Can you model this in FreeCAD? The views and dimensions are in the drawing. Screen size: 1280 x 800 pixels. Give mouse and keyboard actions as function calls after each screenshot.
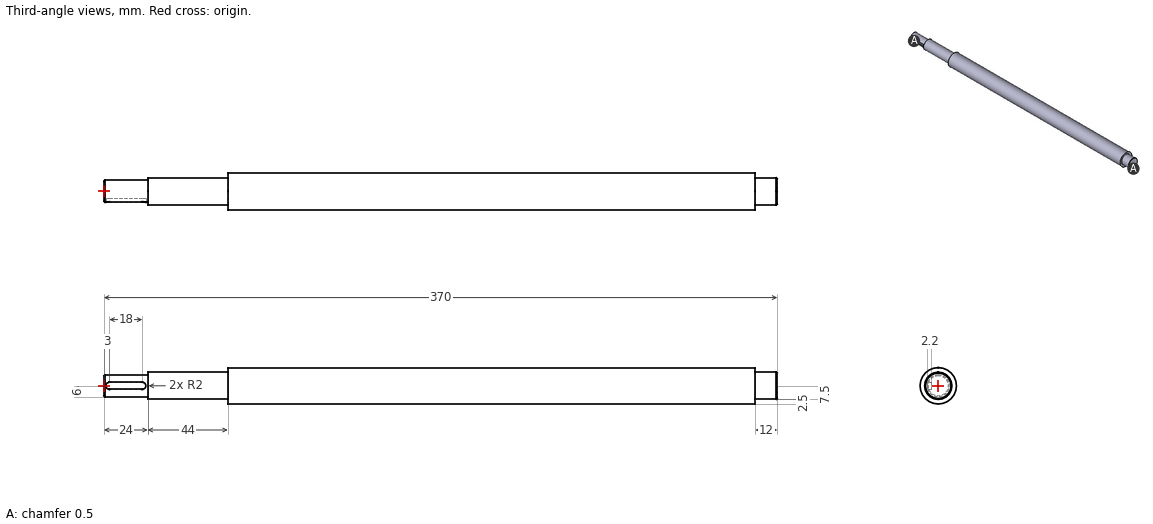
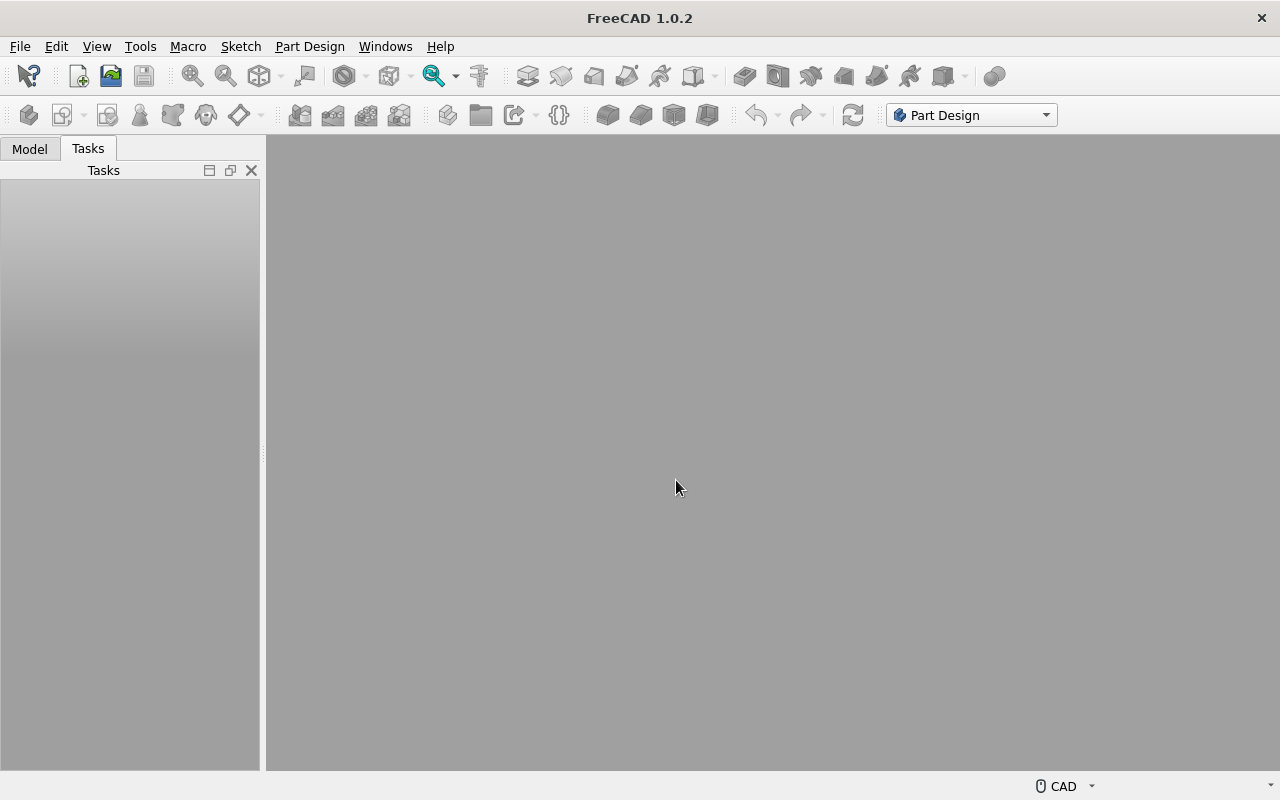
click(78, 76)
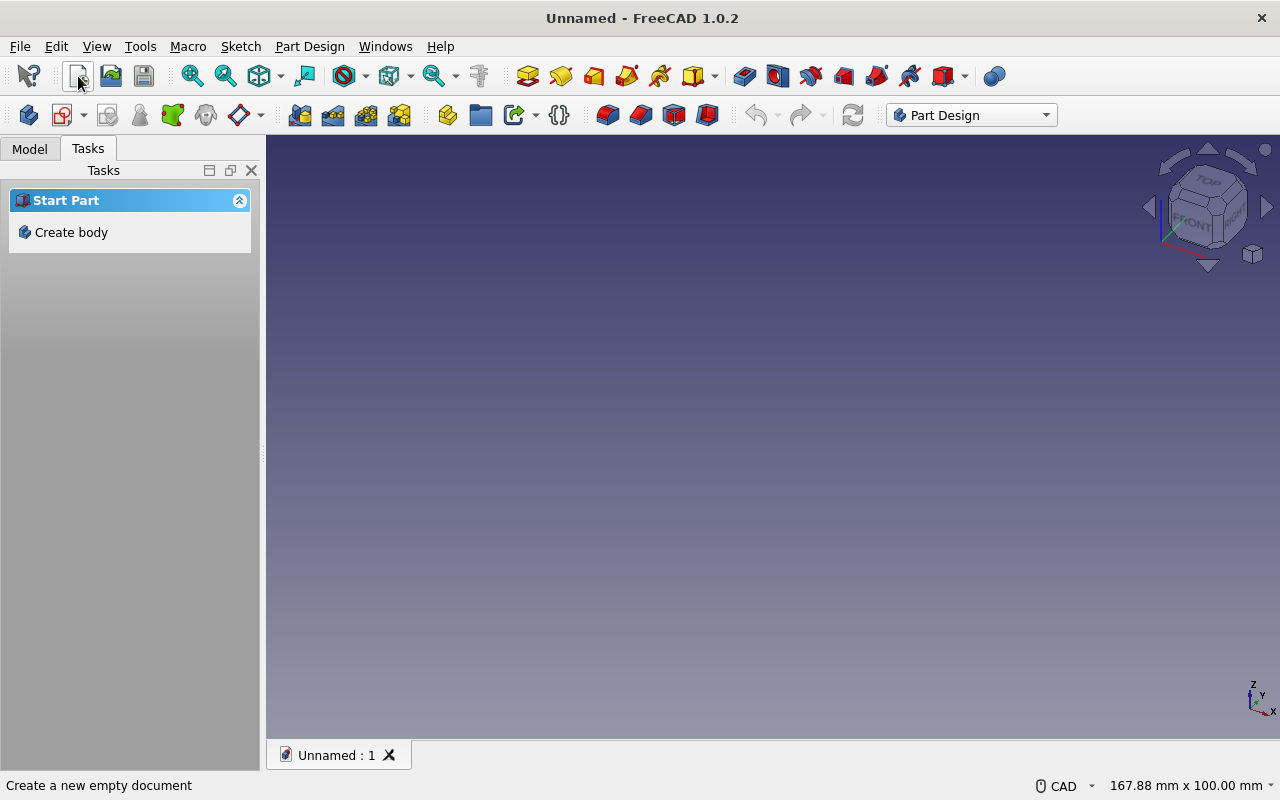
click(62, 116)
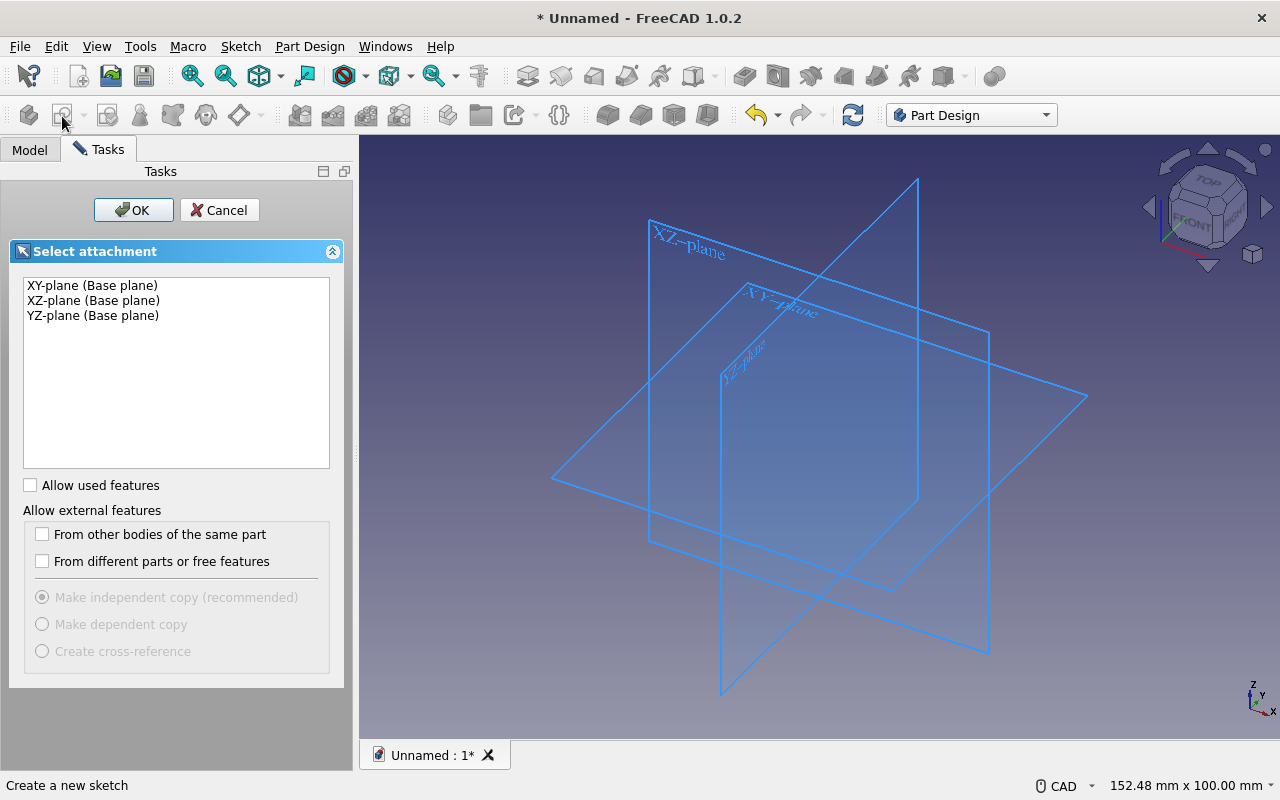
click(84, 300)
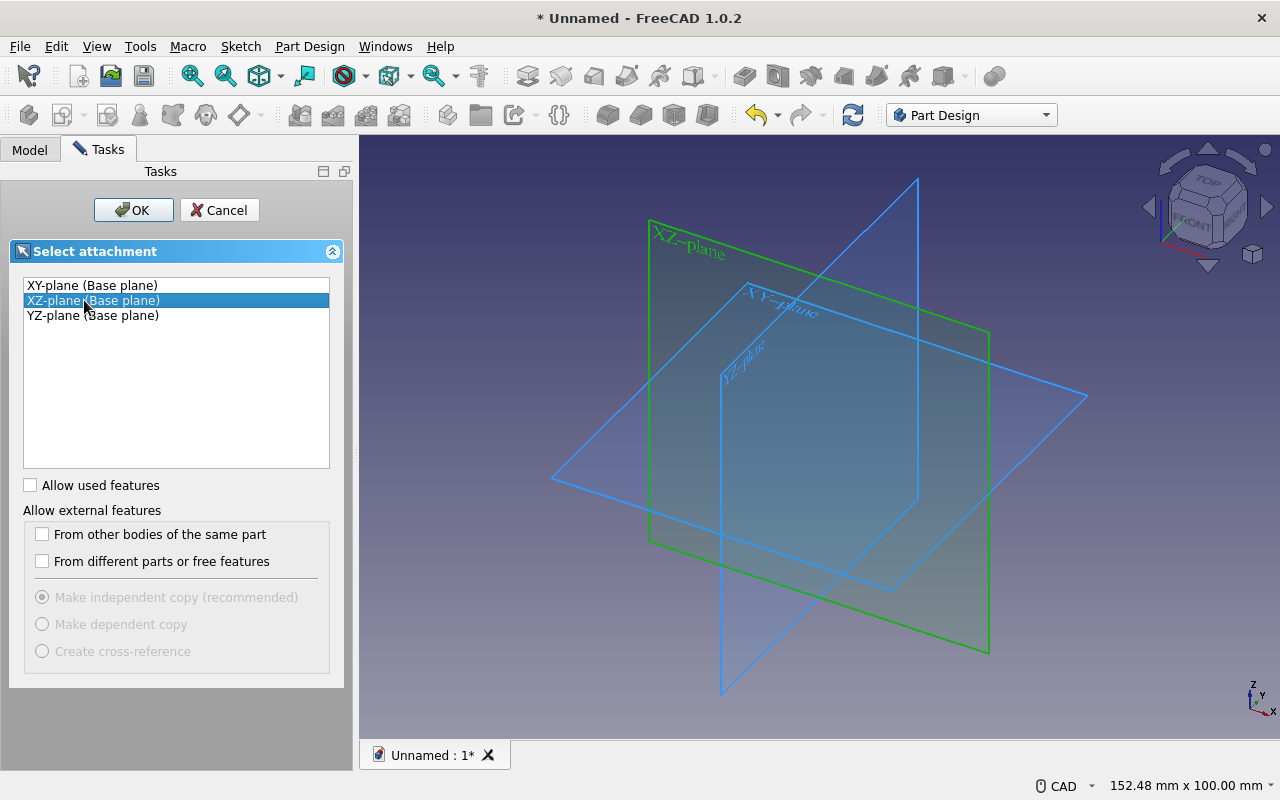
click(134, 210)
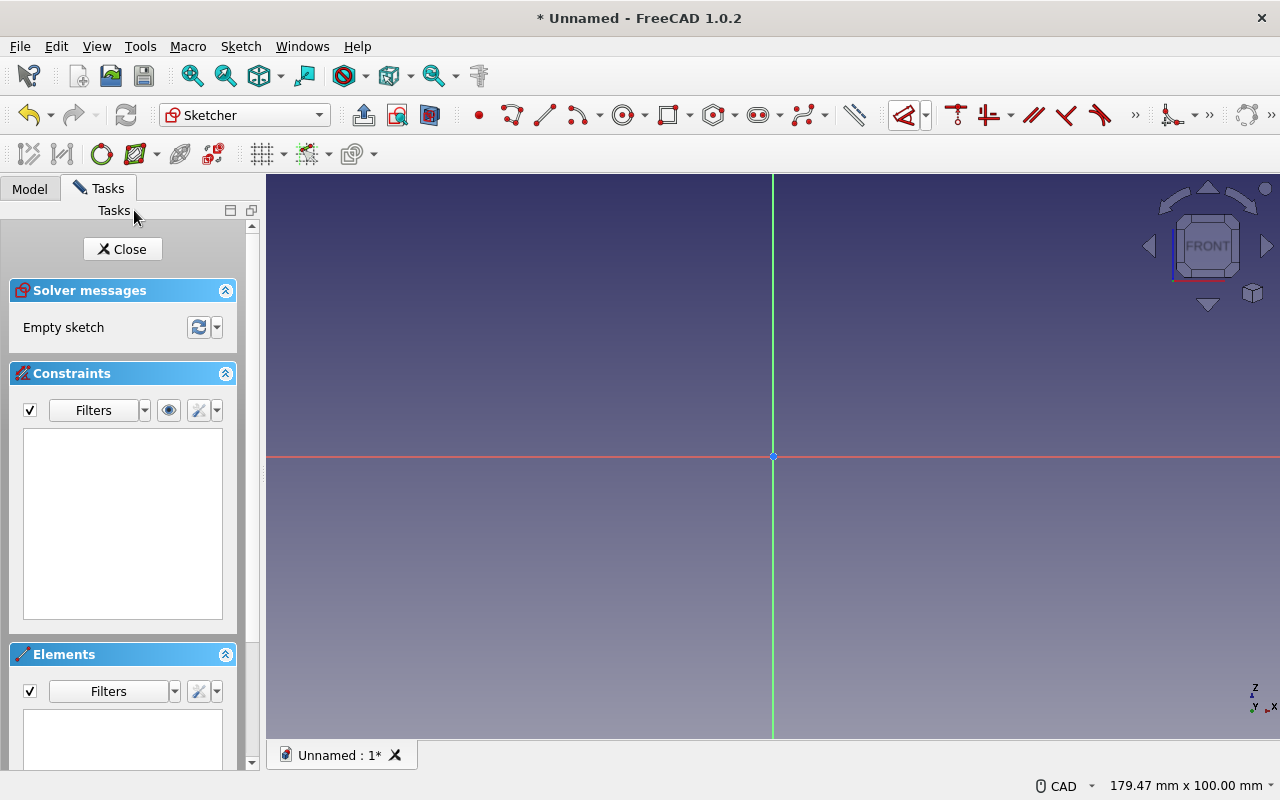
scroll(294, 444, down, 6)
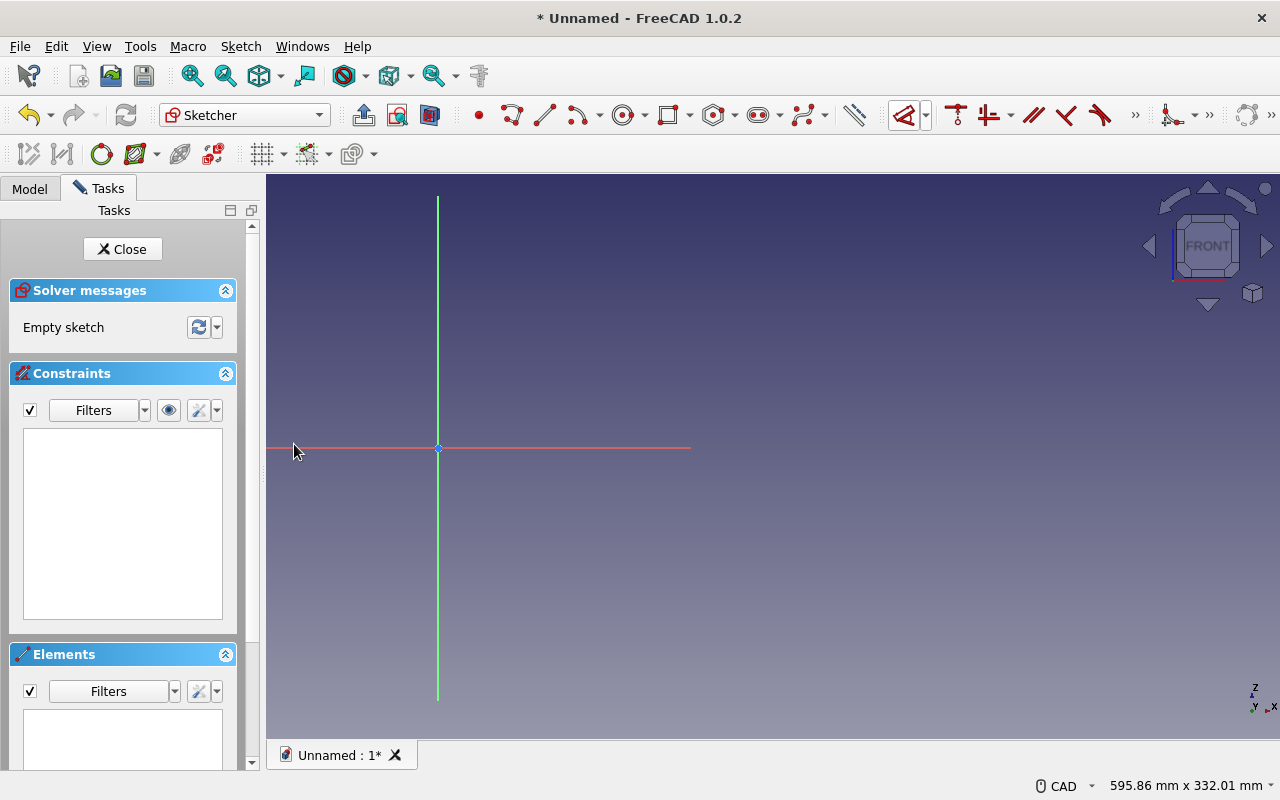
click(512, 116)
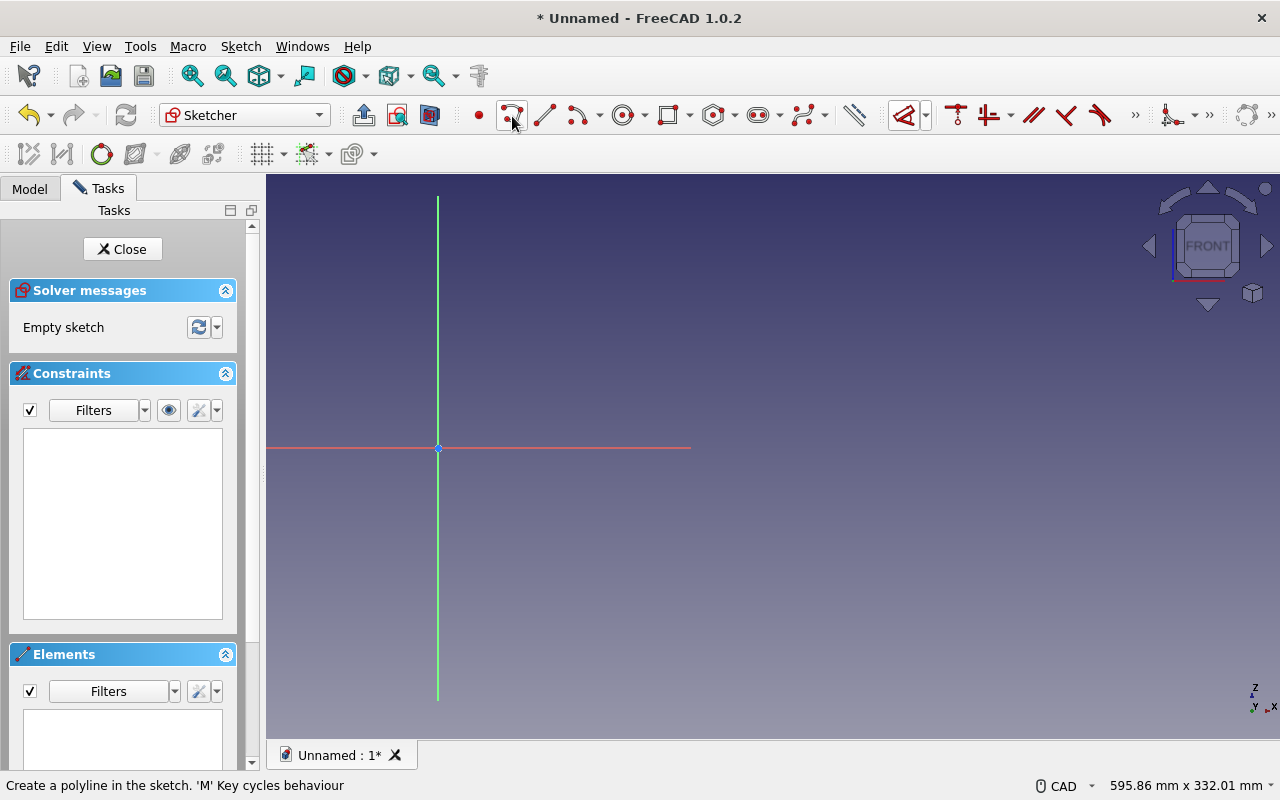
click(438, 448)
click(1068, 457)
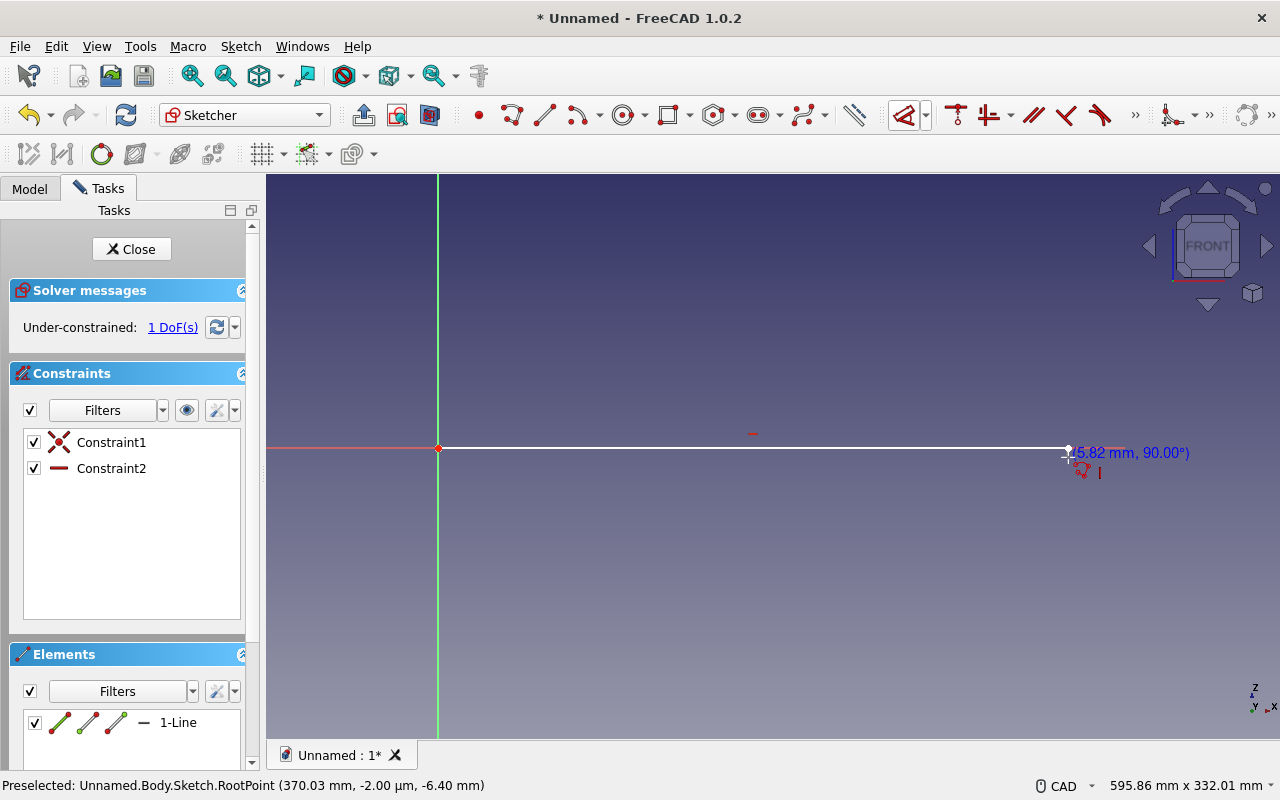
scroll(1068, 461, up, 2)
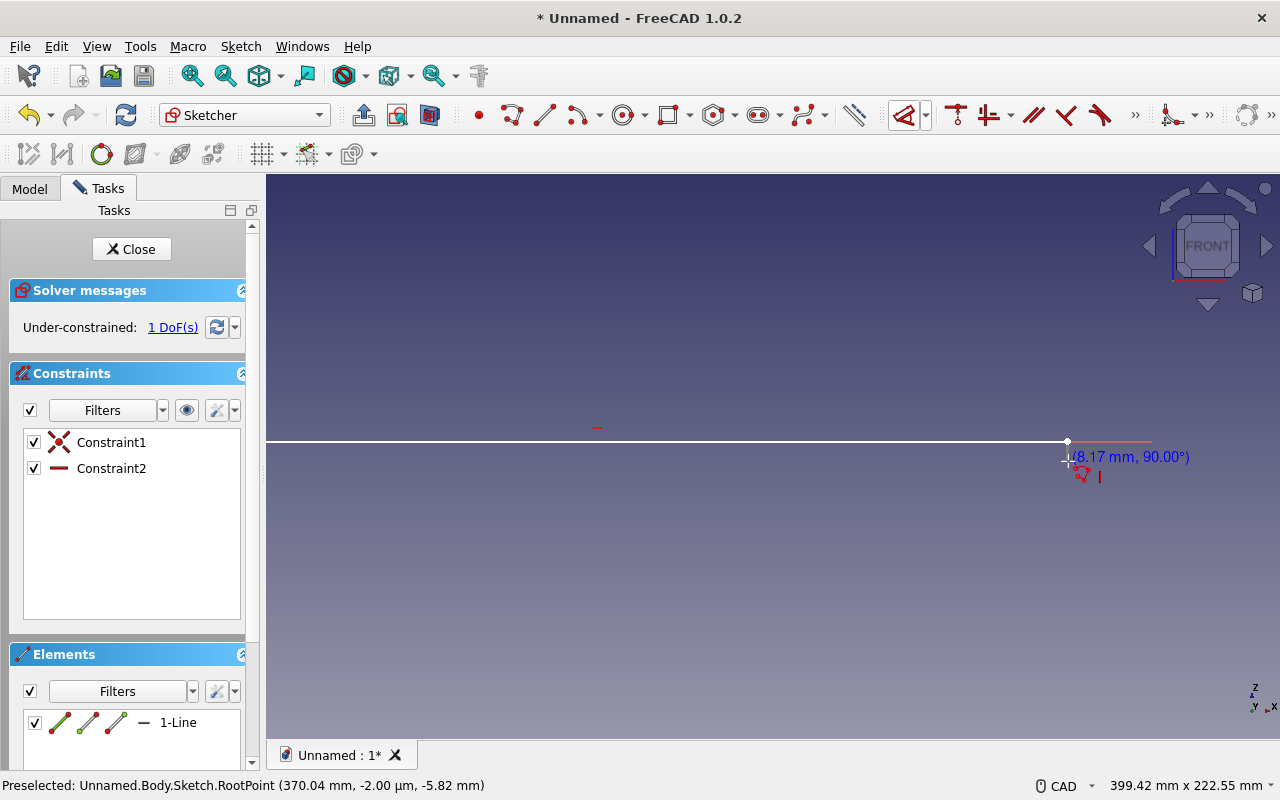
click(1068, 461)
click(1037, 461)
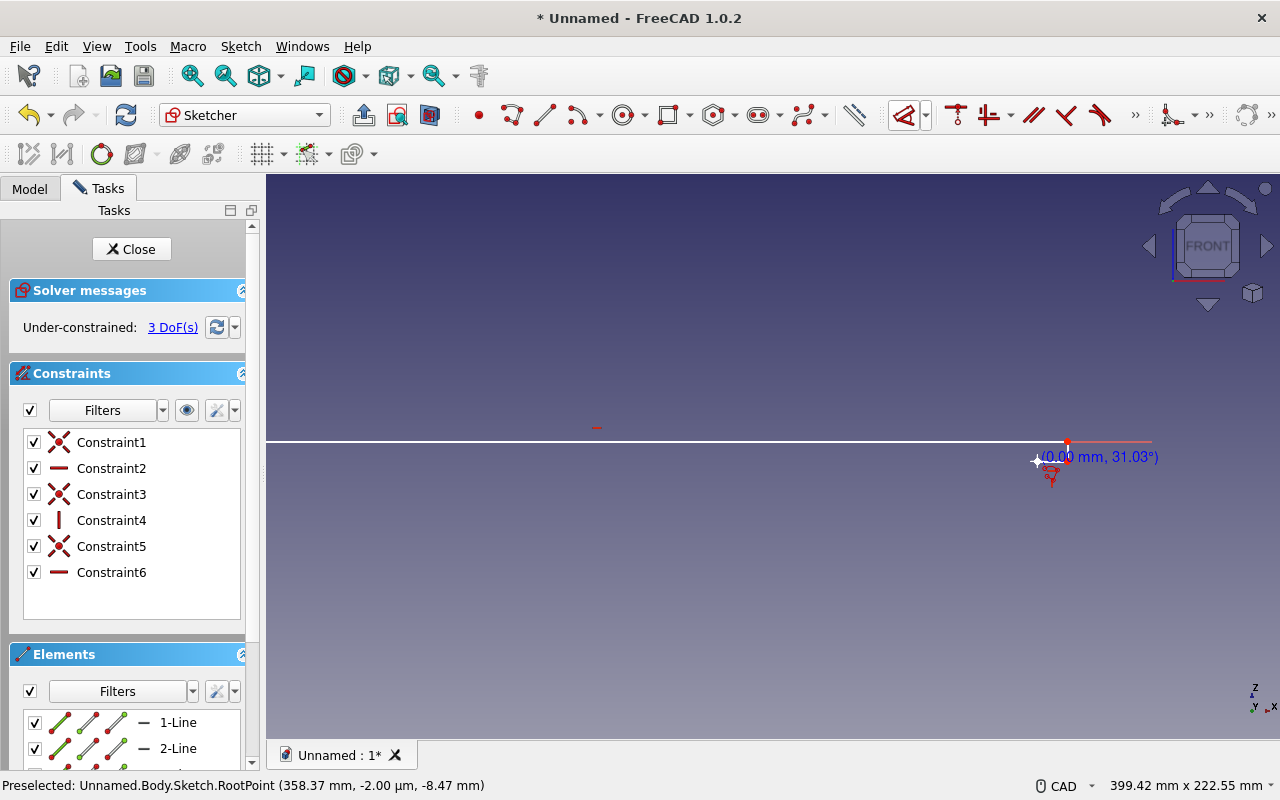
scroll(1037, 467, up, 5)